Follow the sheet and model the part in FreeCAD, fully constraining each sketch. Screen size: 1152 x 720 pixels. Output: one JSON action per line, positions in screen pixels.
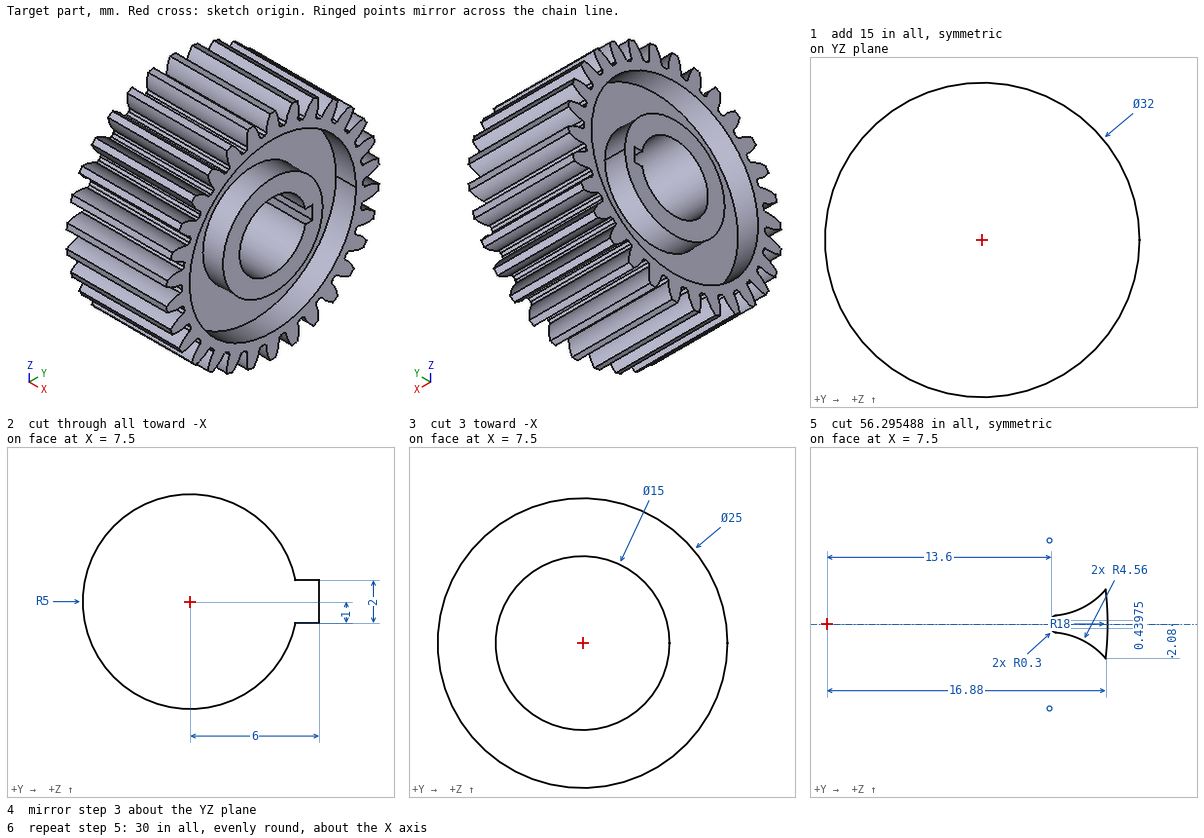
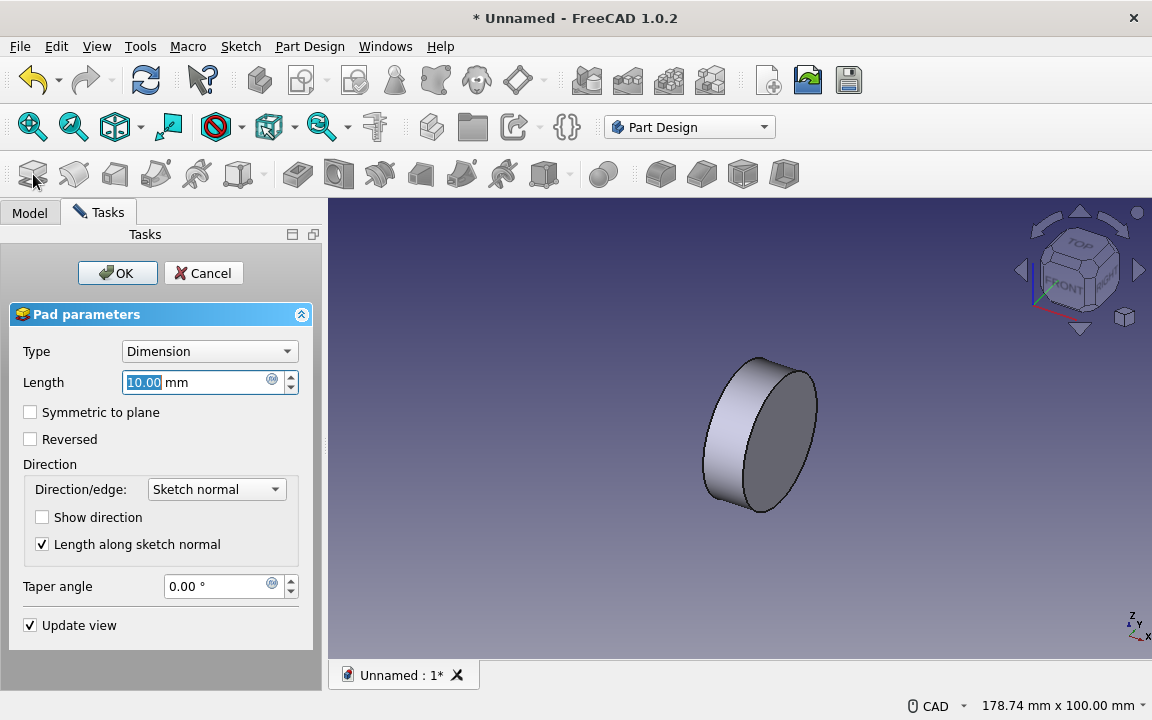
{"action": "type", "text": "15"}
{"action": "key", "text": "Tab"}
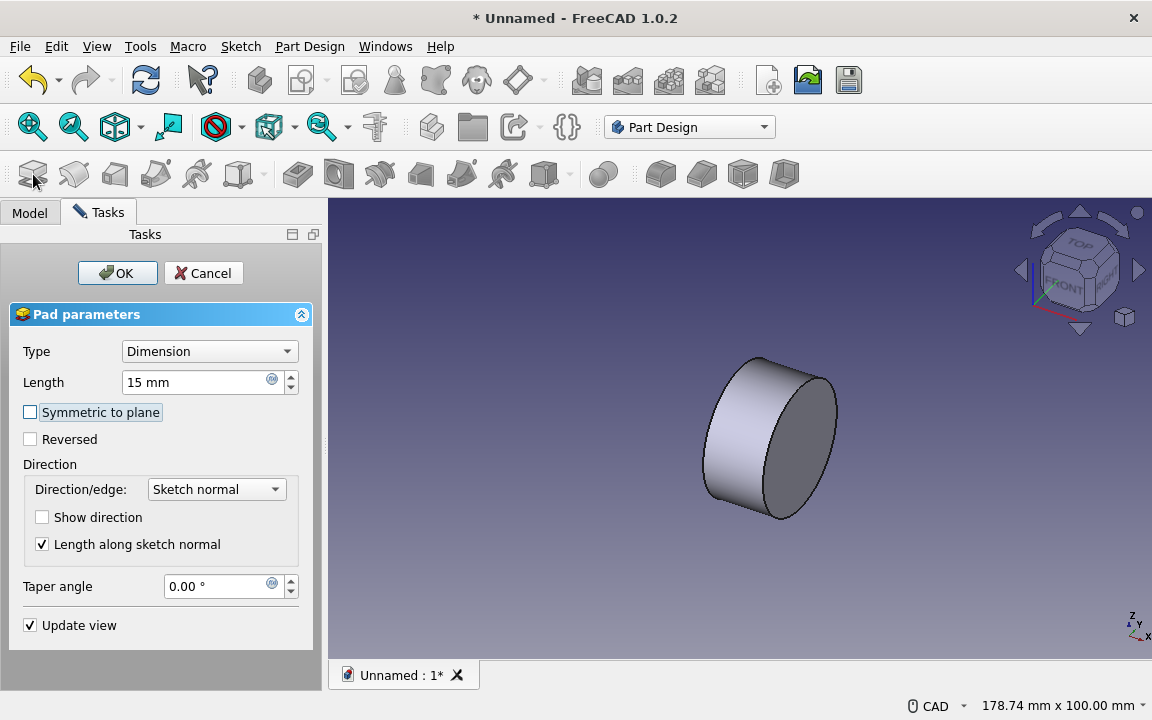
{"action": "left_click", "coordinate": [31, 412]}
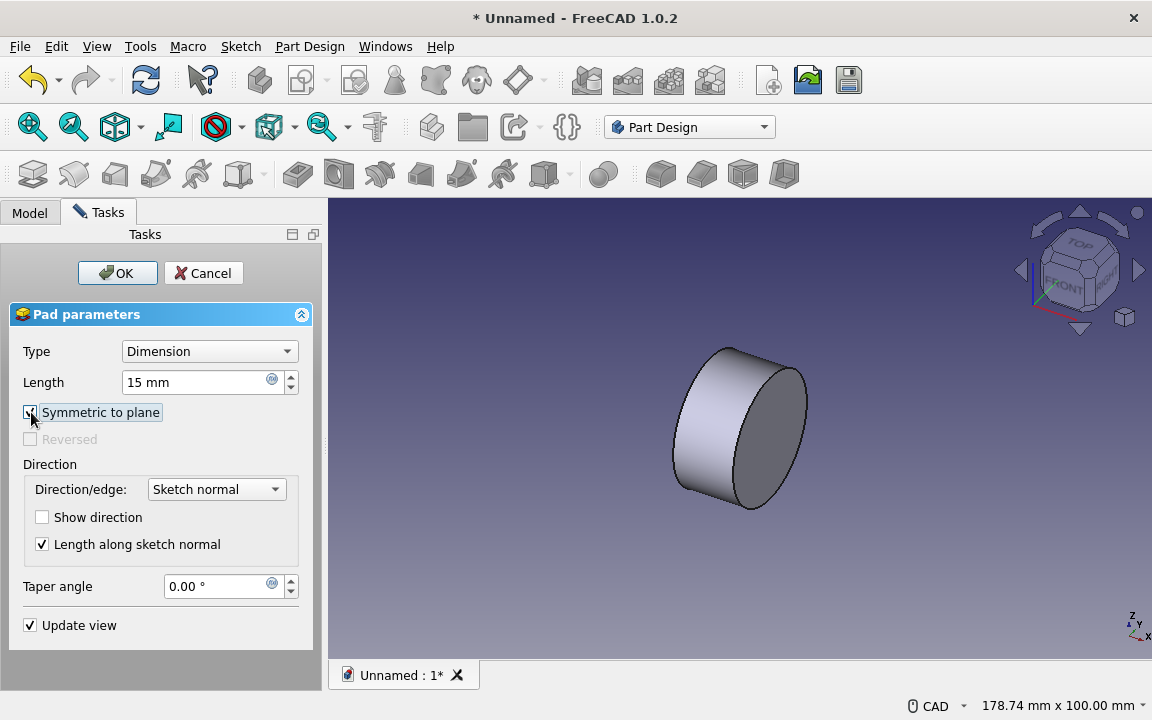
{"action": "left_click", "coordinate": [118, 273]}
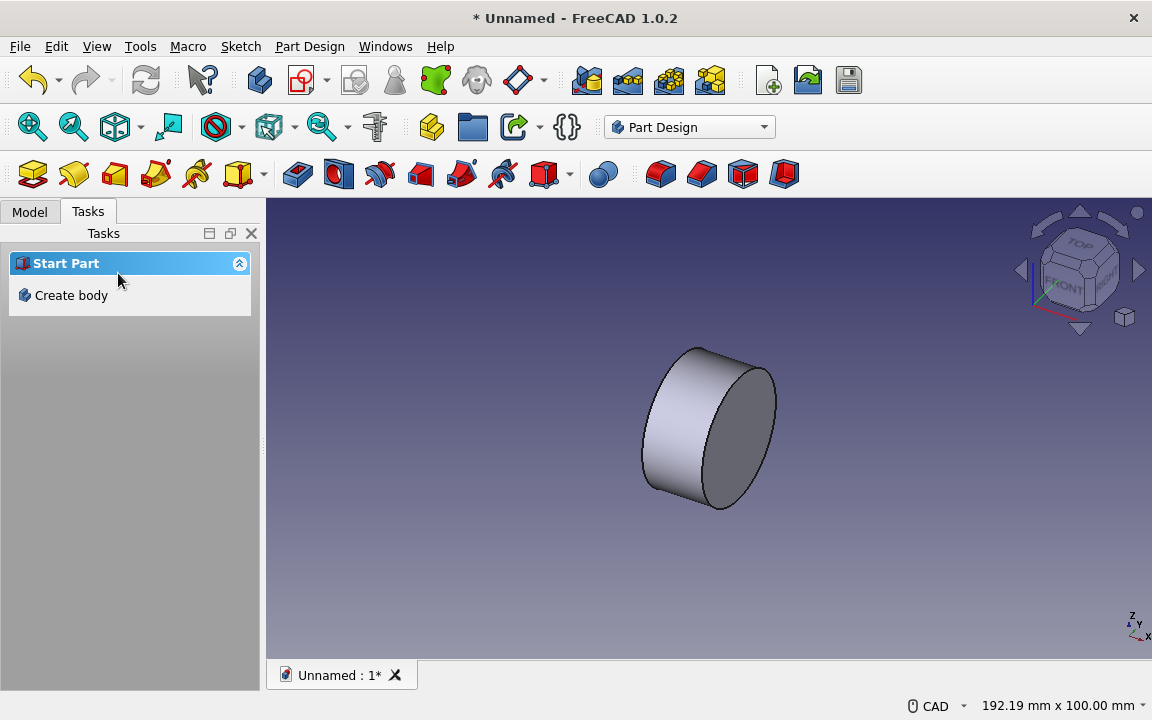
{"action": "left_click", "coordinate": [739, 437]}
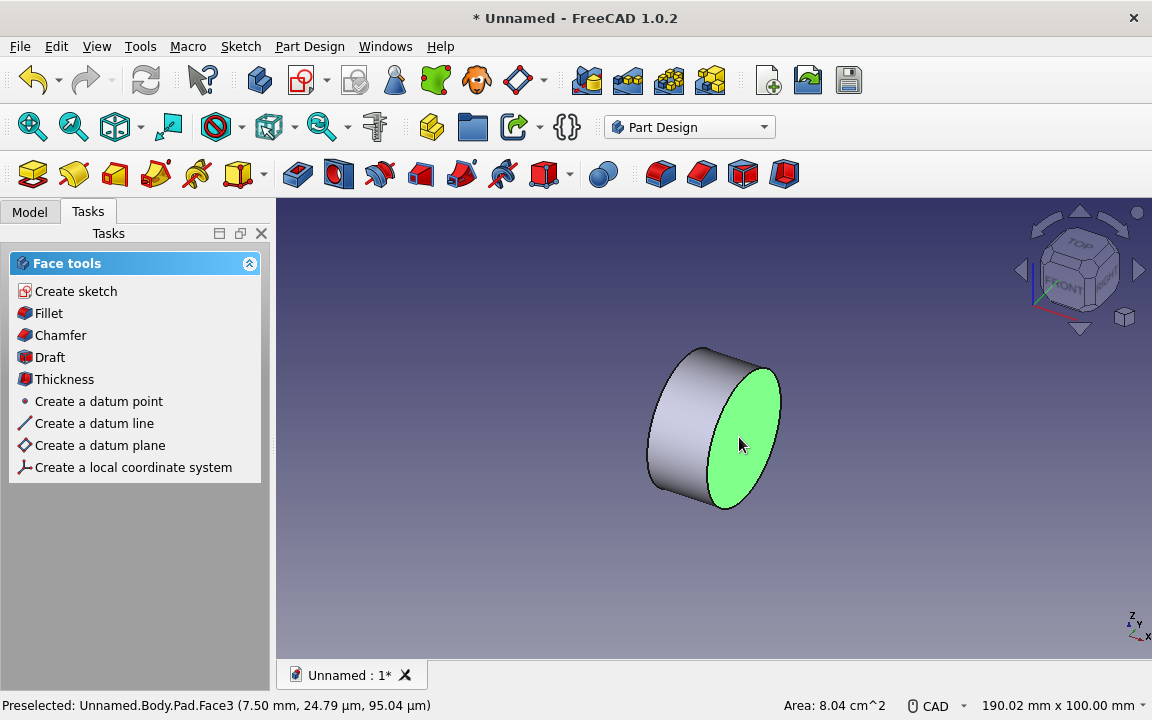
{"action": "left_click", "coordinate": [300, 80]}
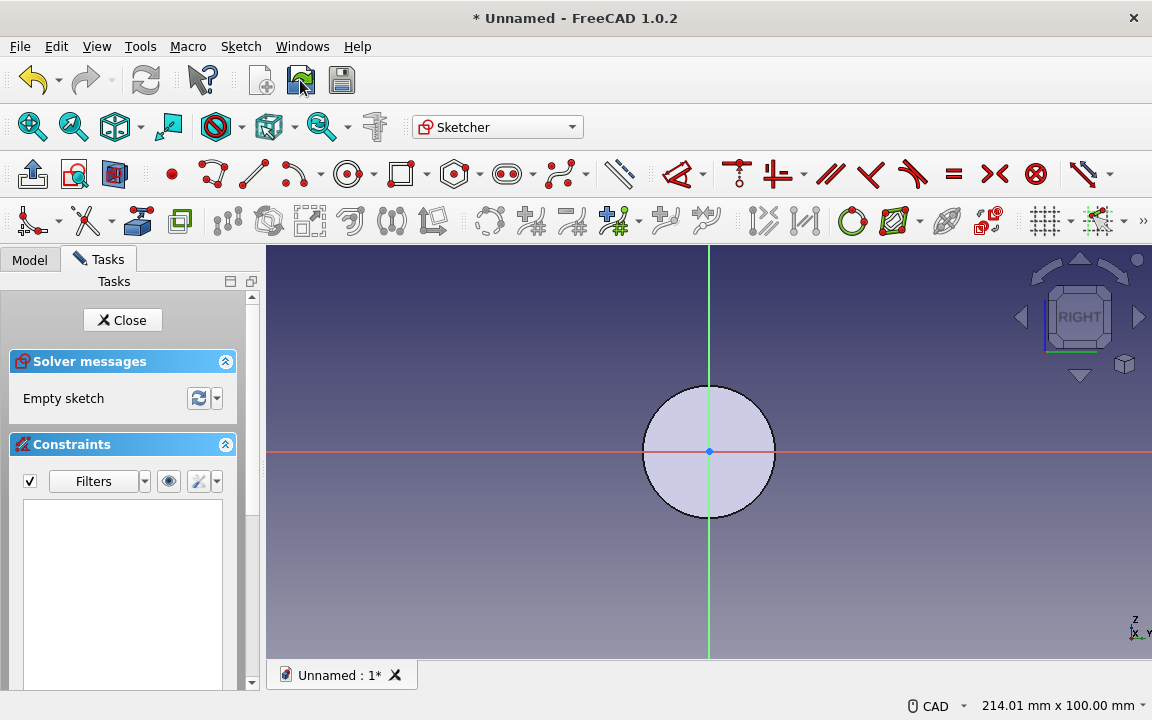
{"action": "scroll", "coordinate": [718, 452], "scroll_direction": "up", "scroll_amount": 12}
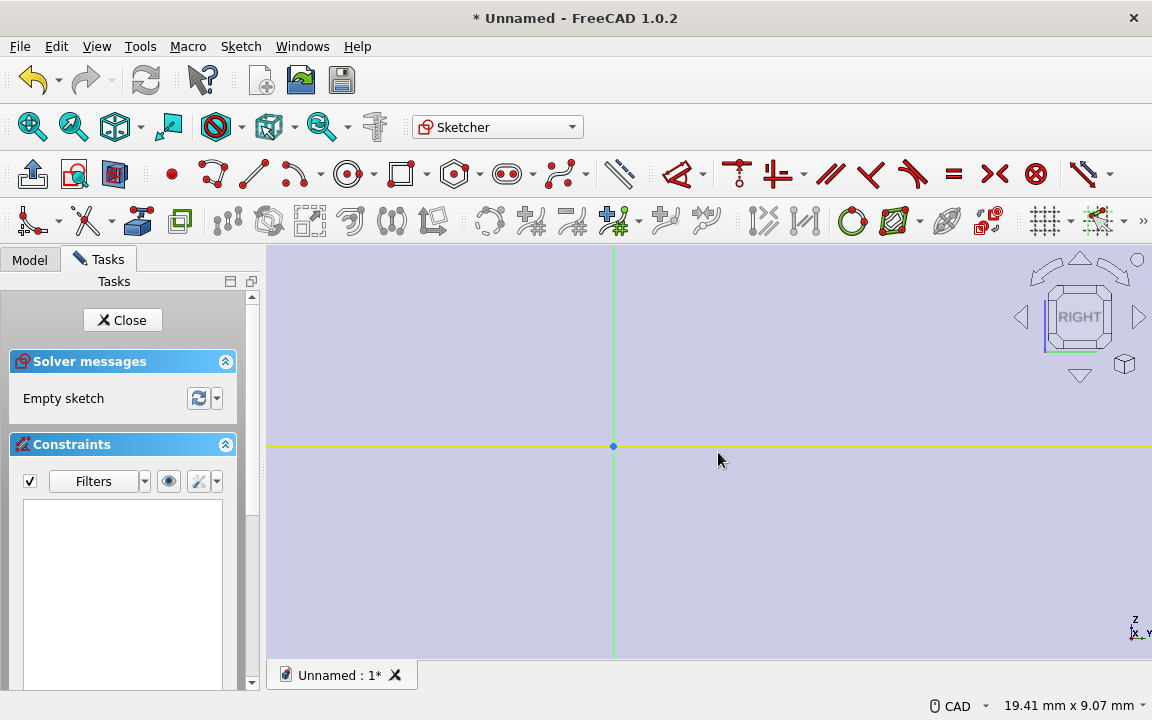
{"action": "left_click", "coordinate": [213, 174]}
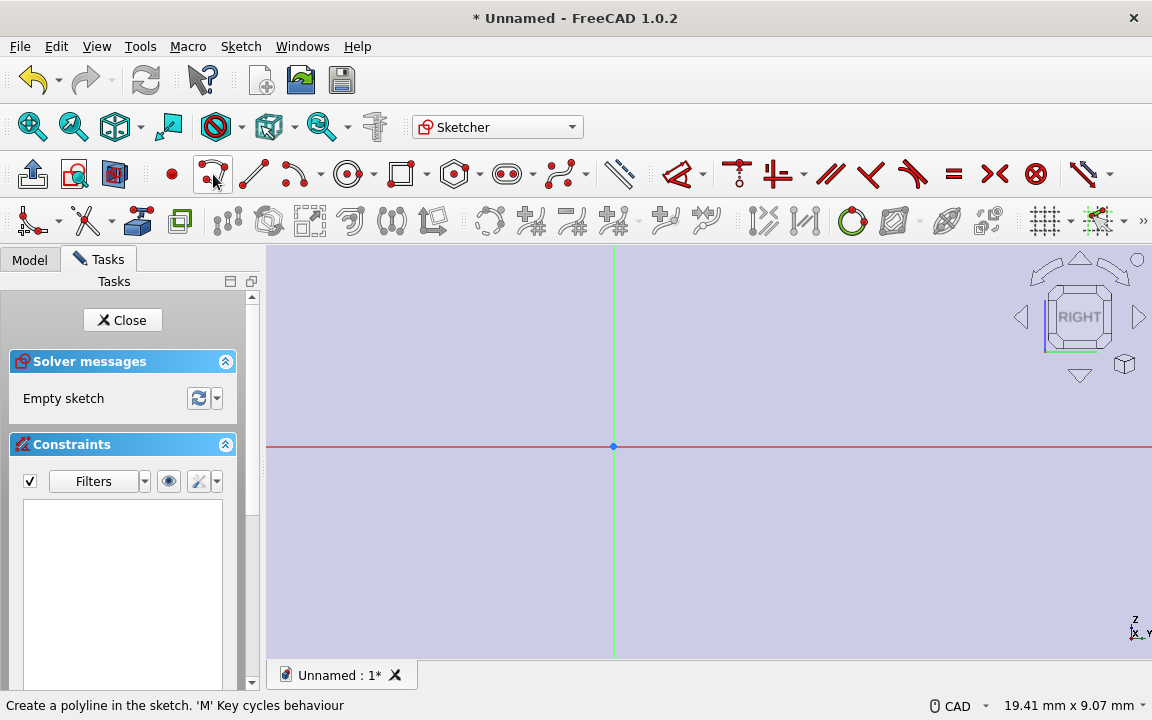
{"action": "left_click", "coordinate": [837, 493]}
{"action": "left_click", "coordinate": [887, 493]}
{"action": "left_click", "coordinate": [887, 401]}
{"action": "left_click", "coordinate": [837, 401]}
{"action": "right_click", "coordinate": [837, 401]}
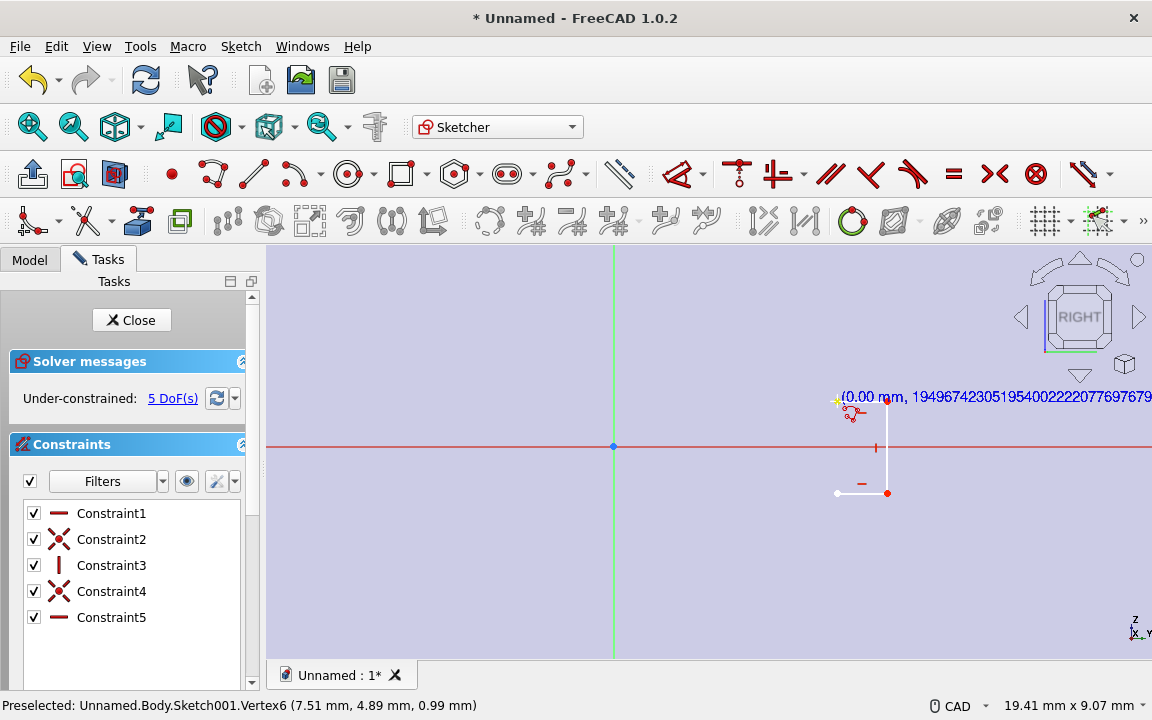
{"action": "key", "text": "g 3 a"}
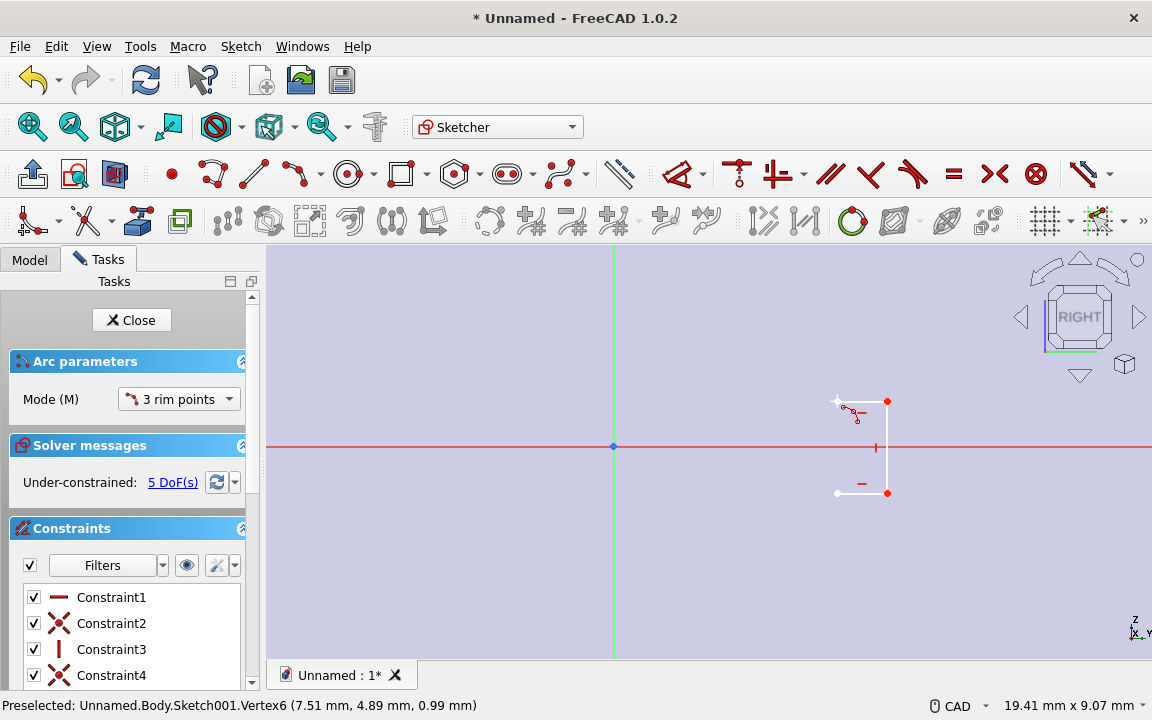
{"action": "left_click", "coordinate": [837, 402]}
{"action": "left_click", "coordinate": [837, 494]}
{"action": "left_click", "coordinate": [424, 320]}
{"action": "key", "text": "Escape"}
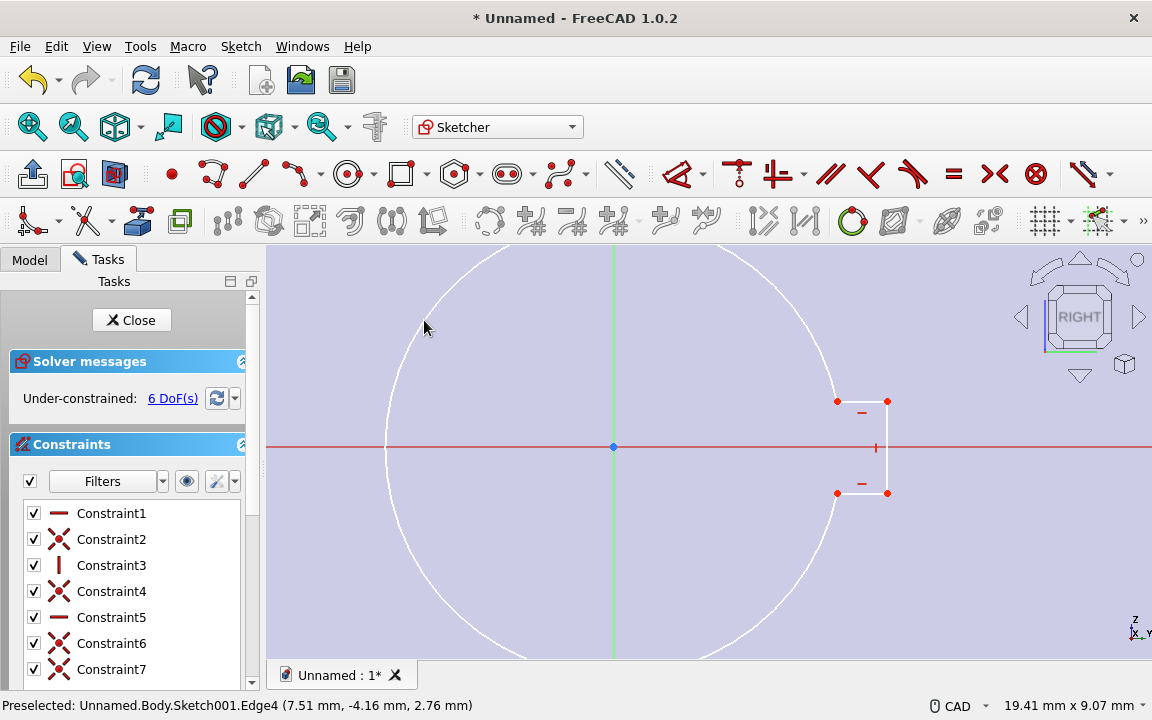
{"action": "left_click_drag", "start_coordinate": [604, 437], "coordinate": [624, 458]}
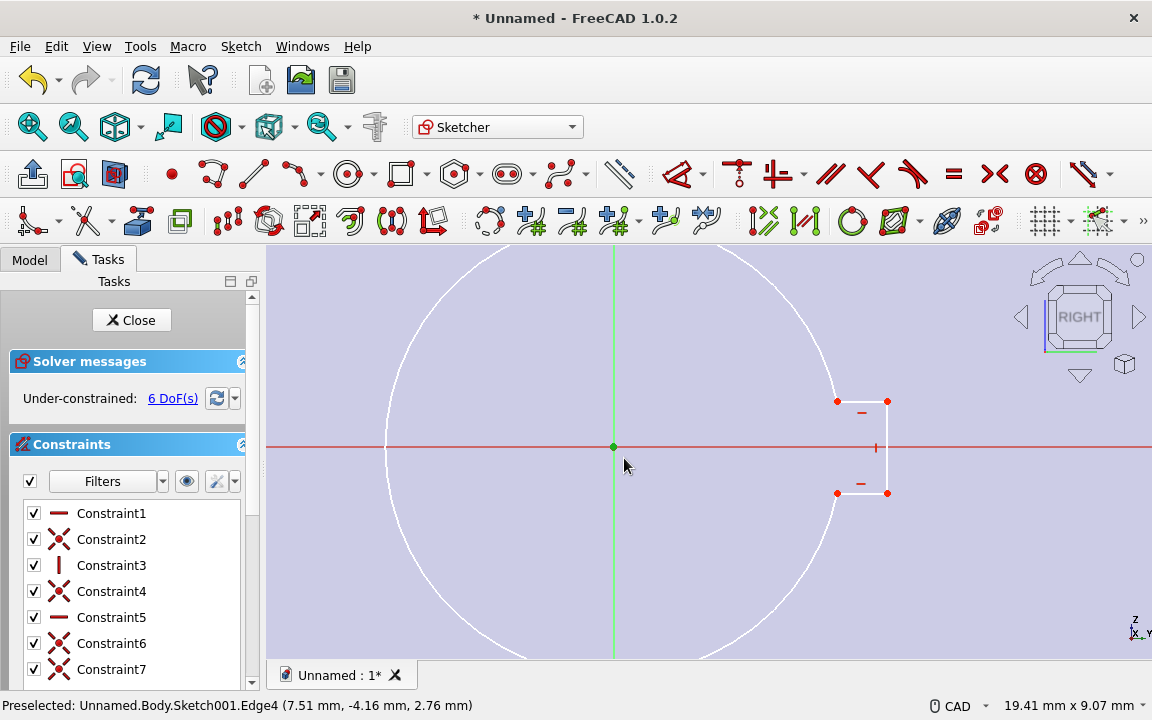
{"action": "key", "text": "c"}